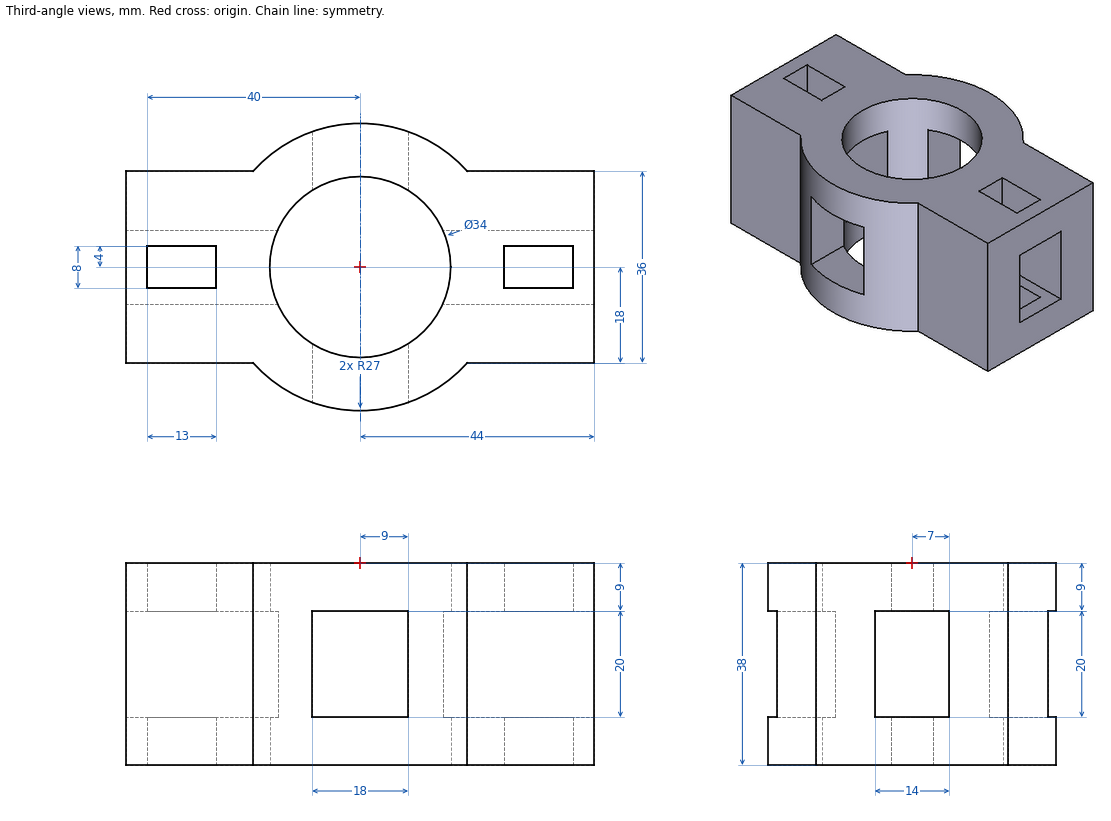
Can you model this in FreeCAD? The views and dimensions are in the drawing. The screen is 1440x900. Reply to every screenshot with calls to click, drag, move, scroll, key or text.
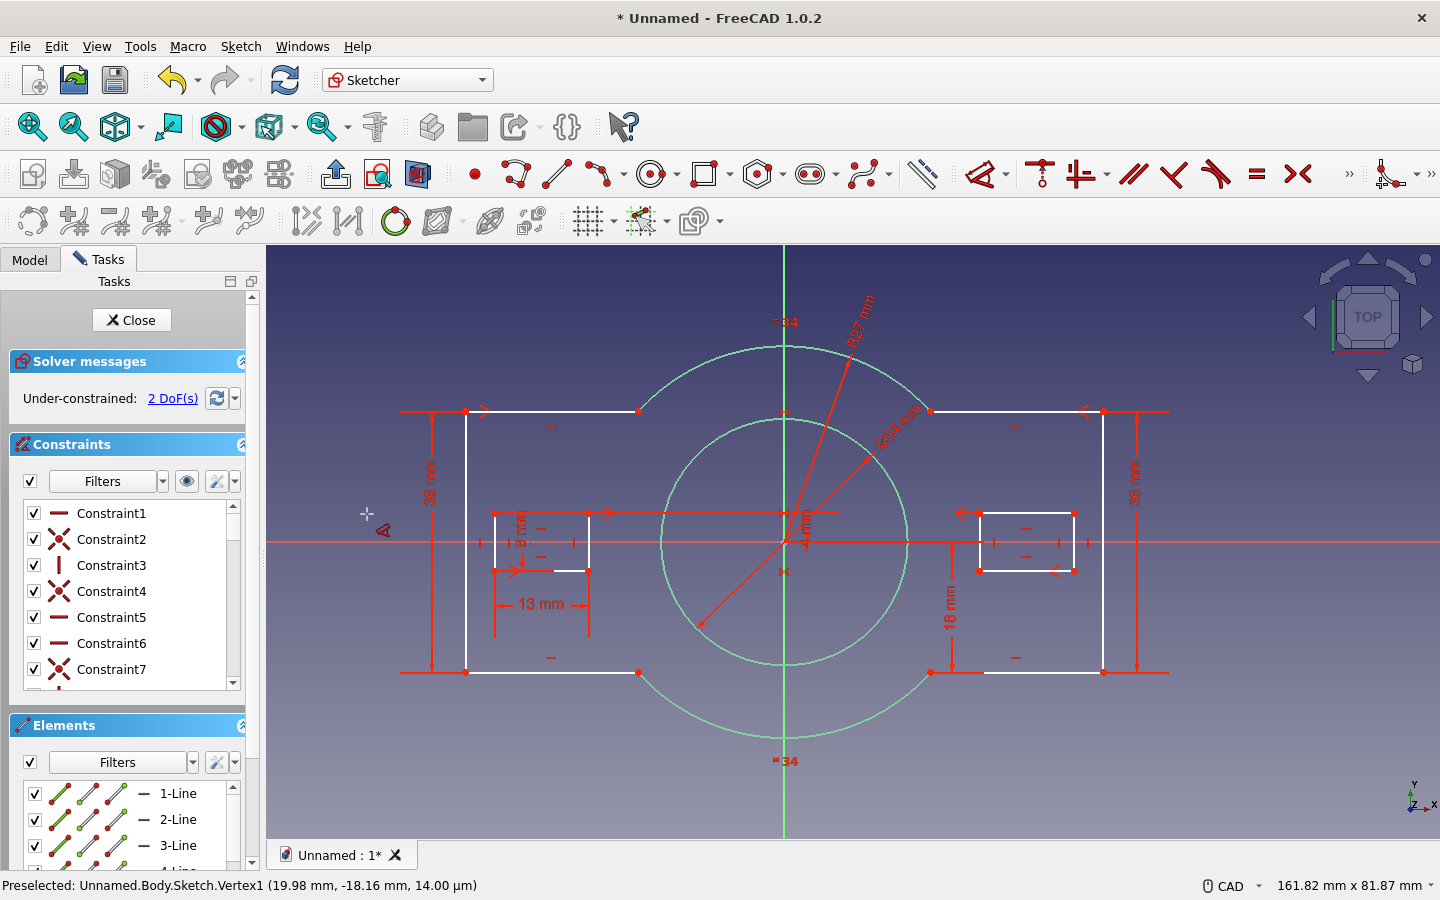
click(1103, 673)
click(944, 707)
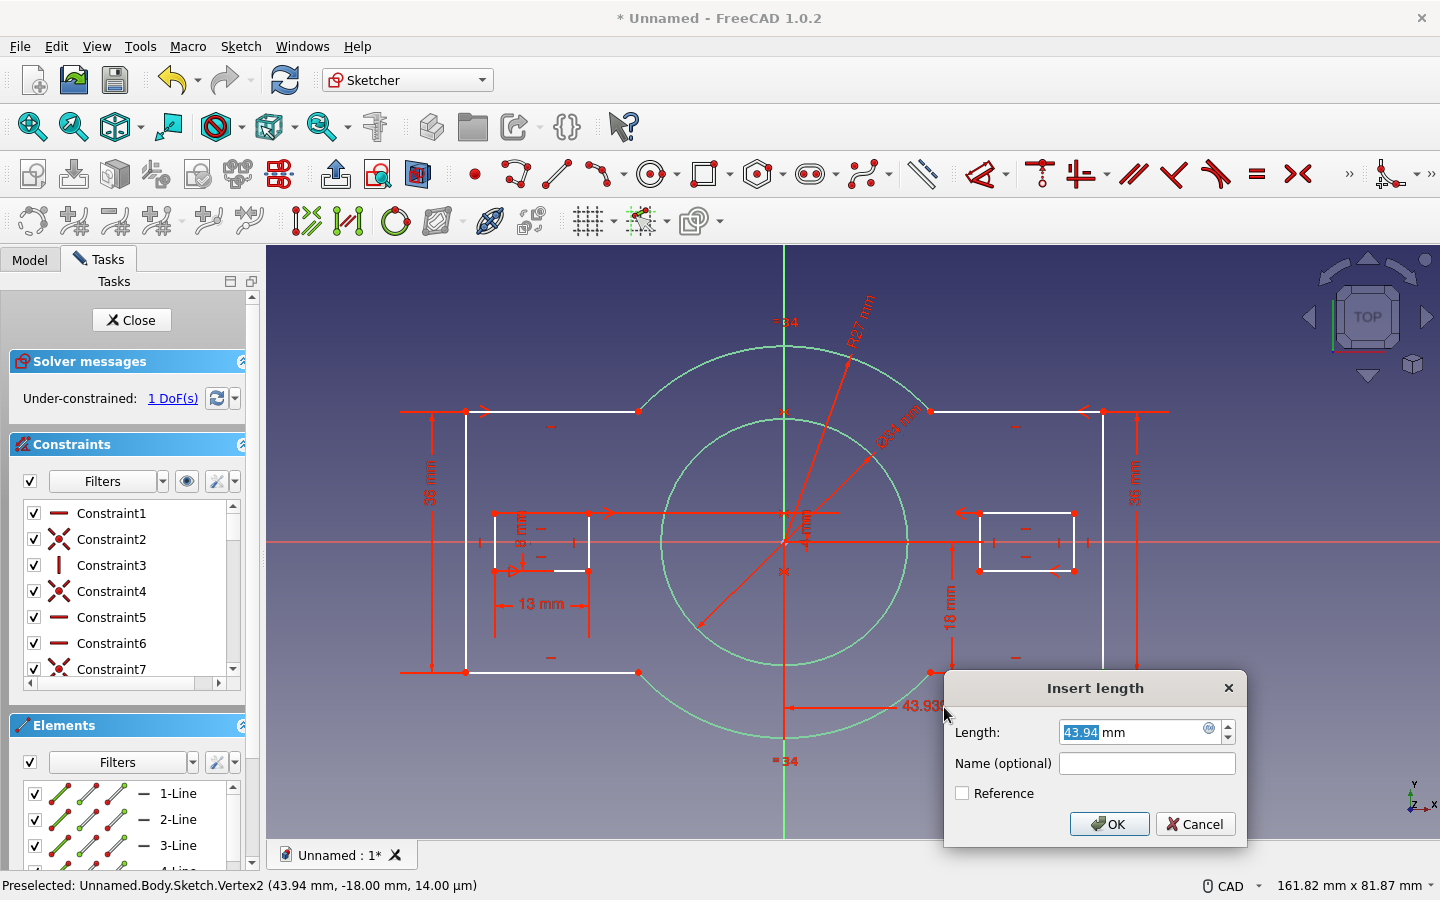
text(44)
key(Return)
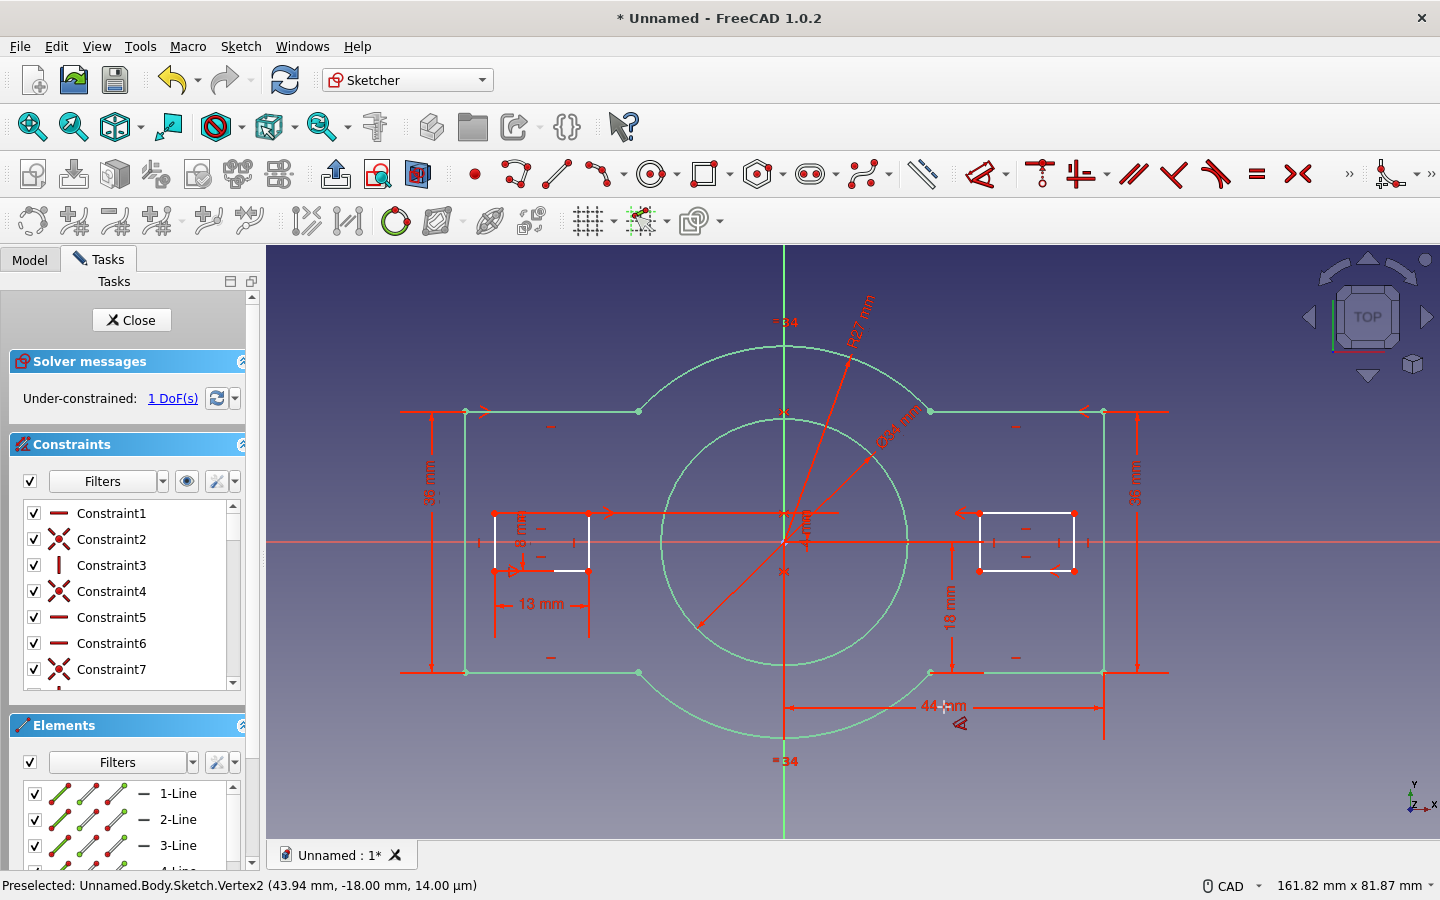
click(495, 513)
click(639, 479)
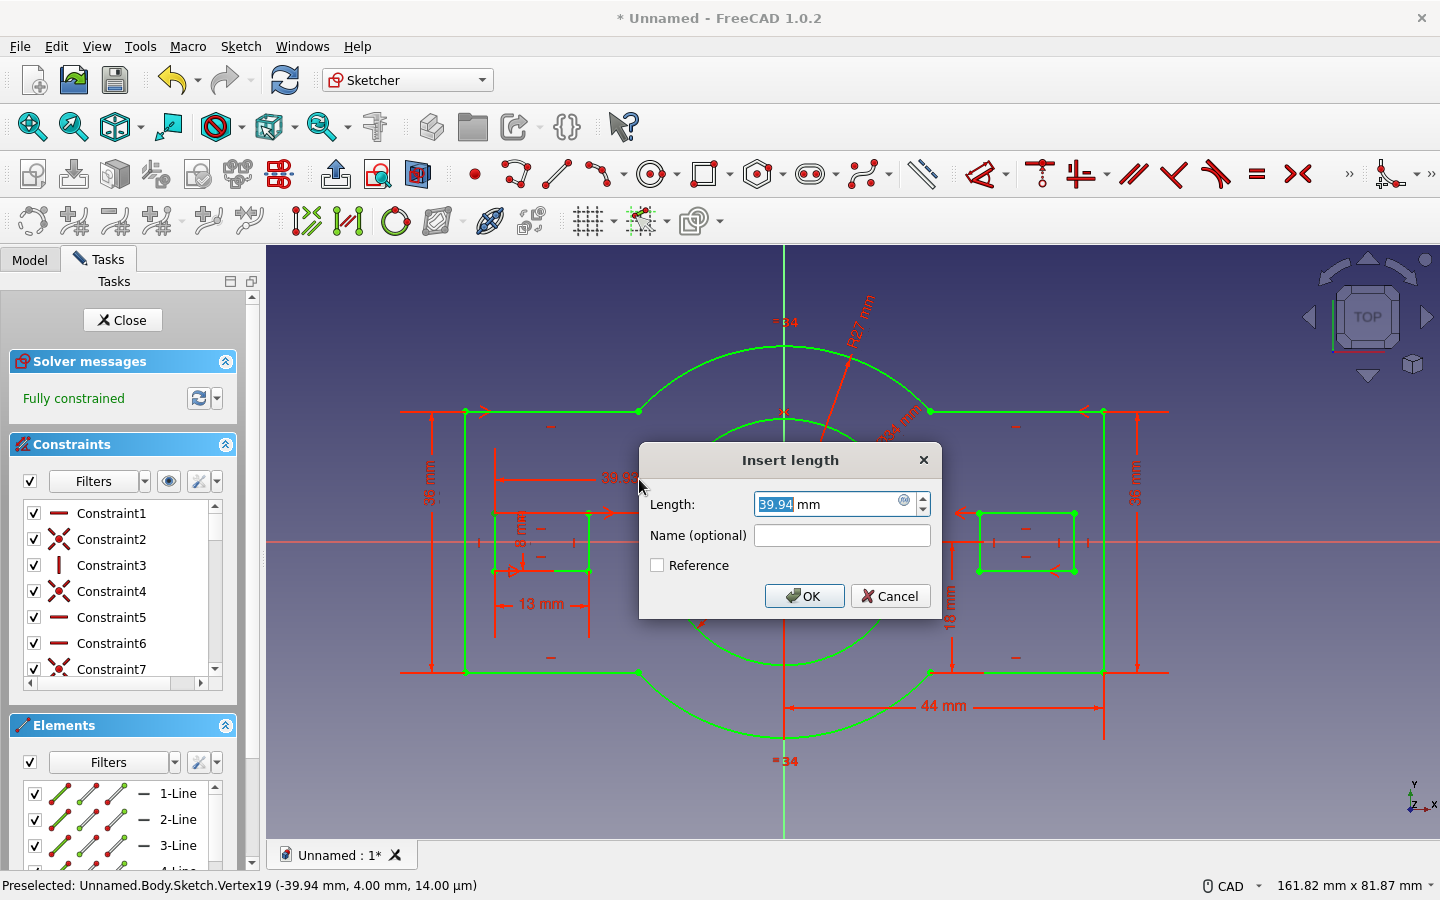
text(40)
key(Return)
key(Escape)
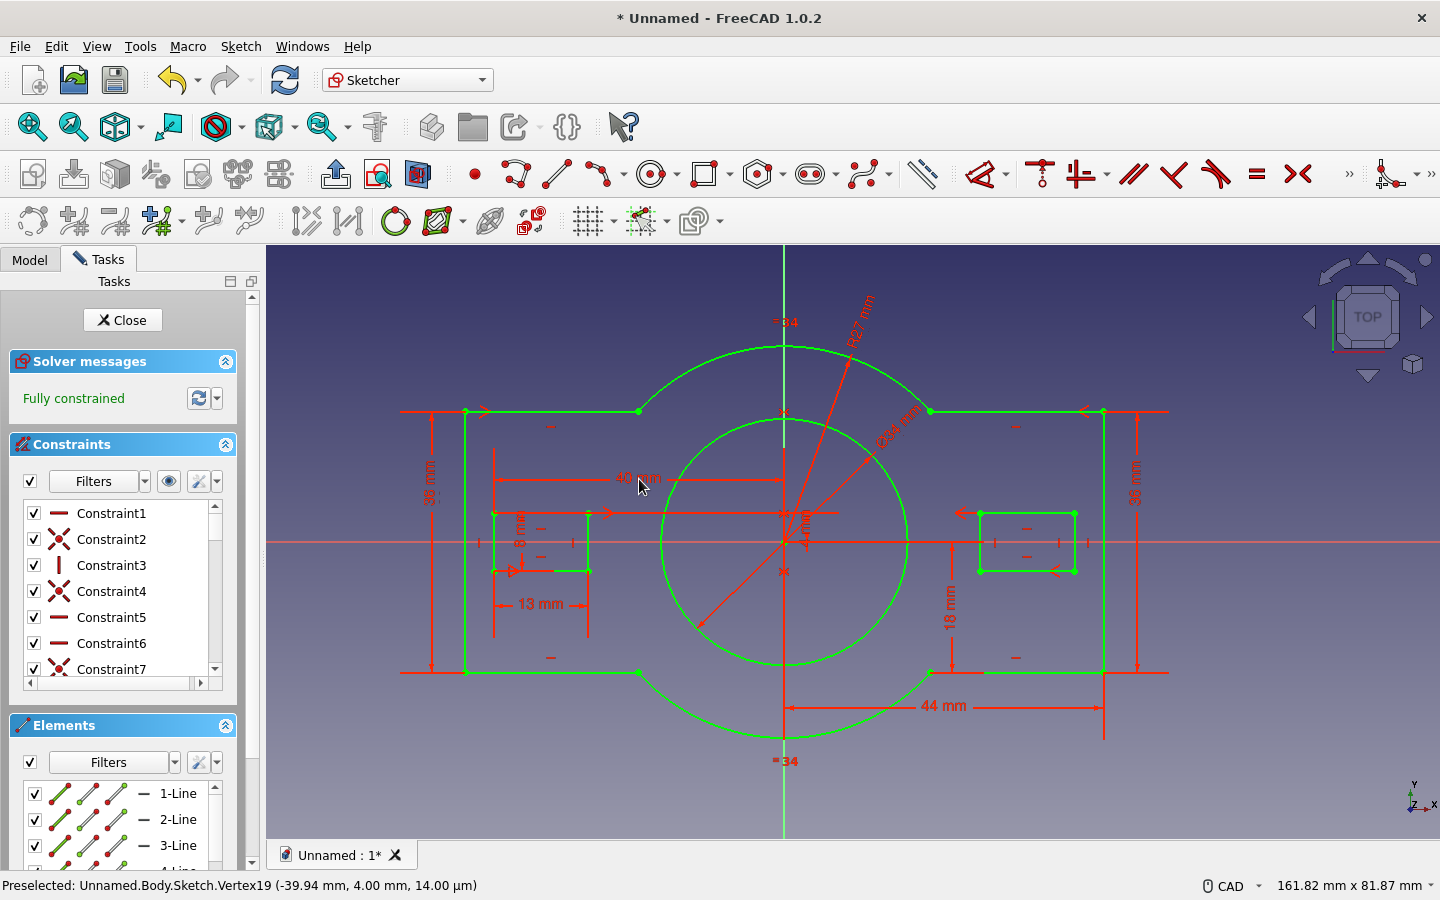
click(123, 320)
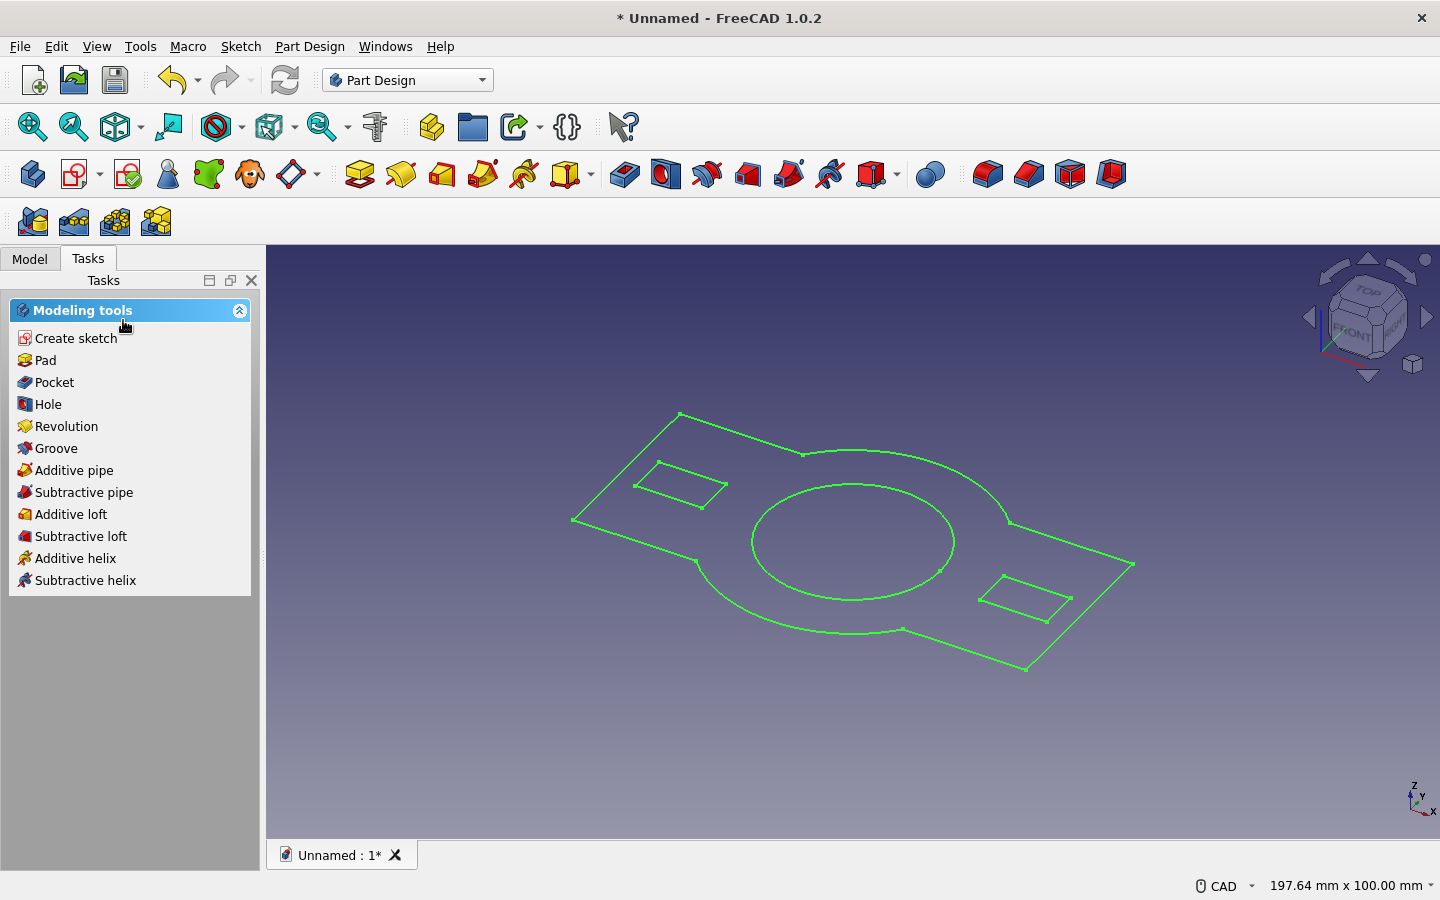
click(360, 174)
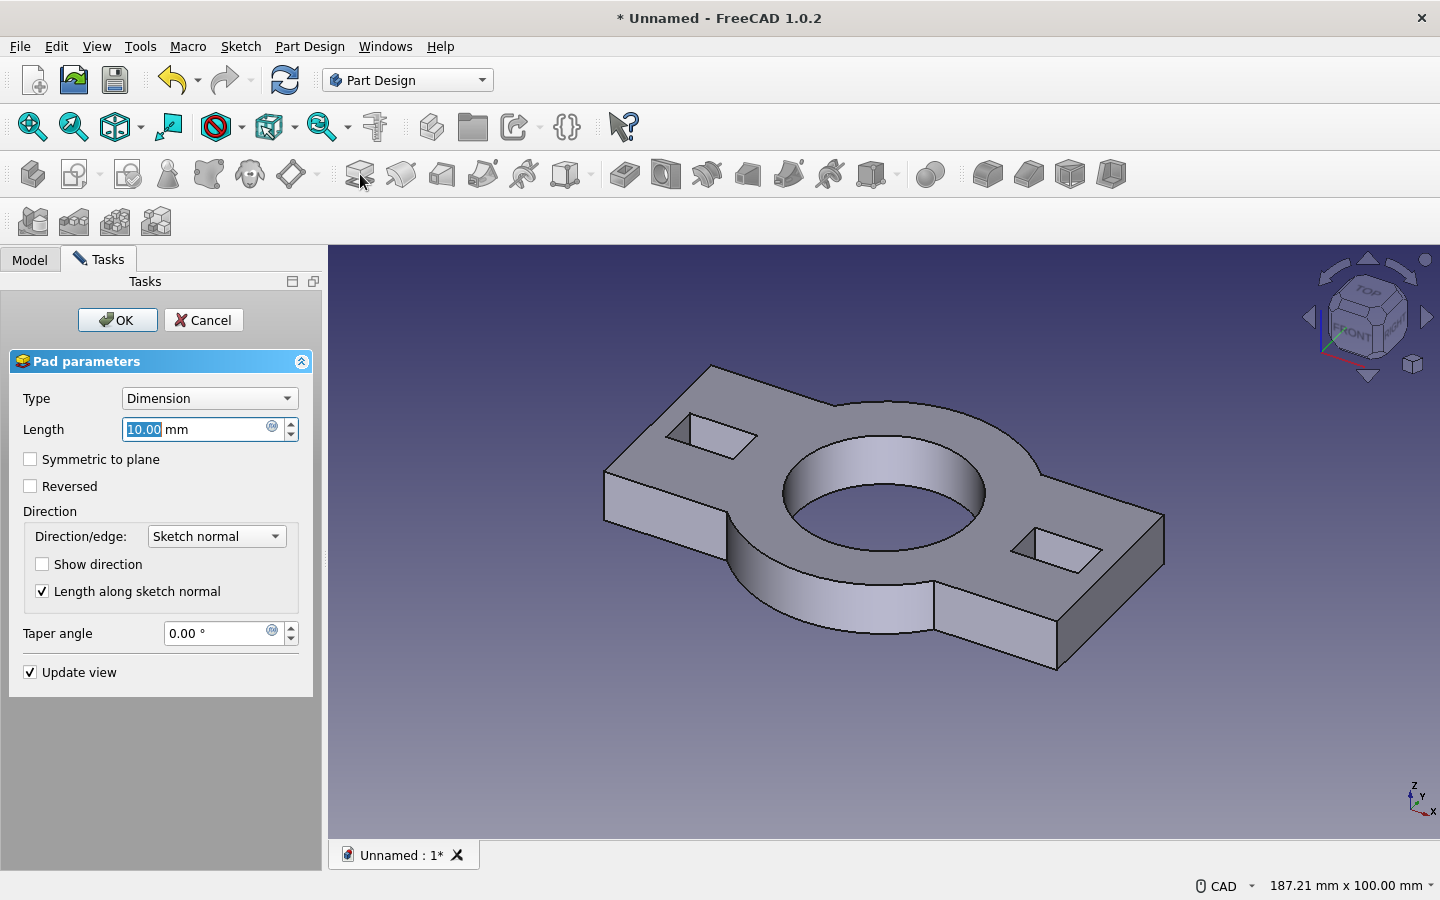
text(38)
key(Tab)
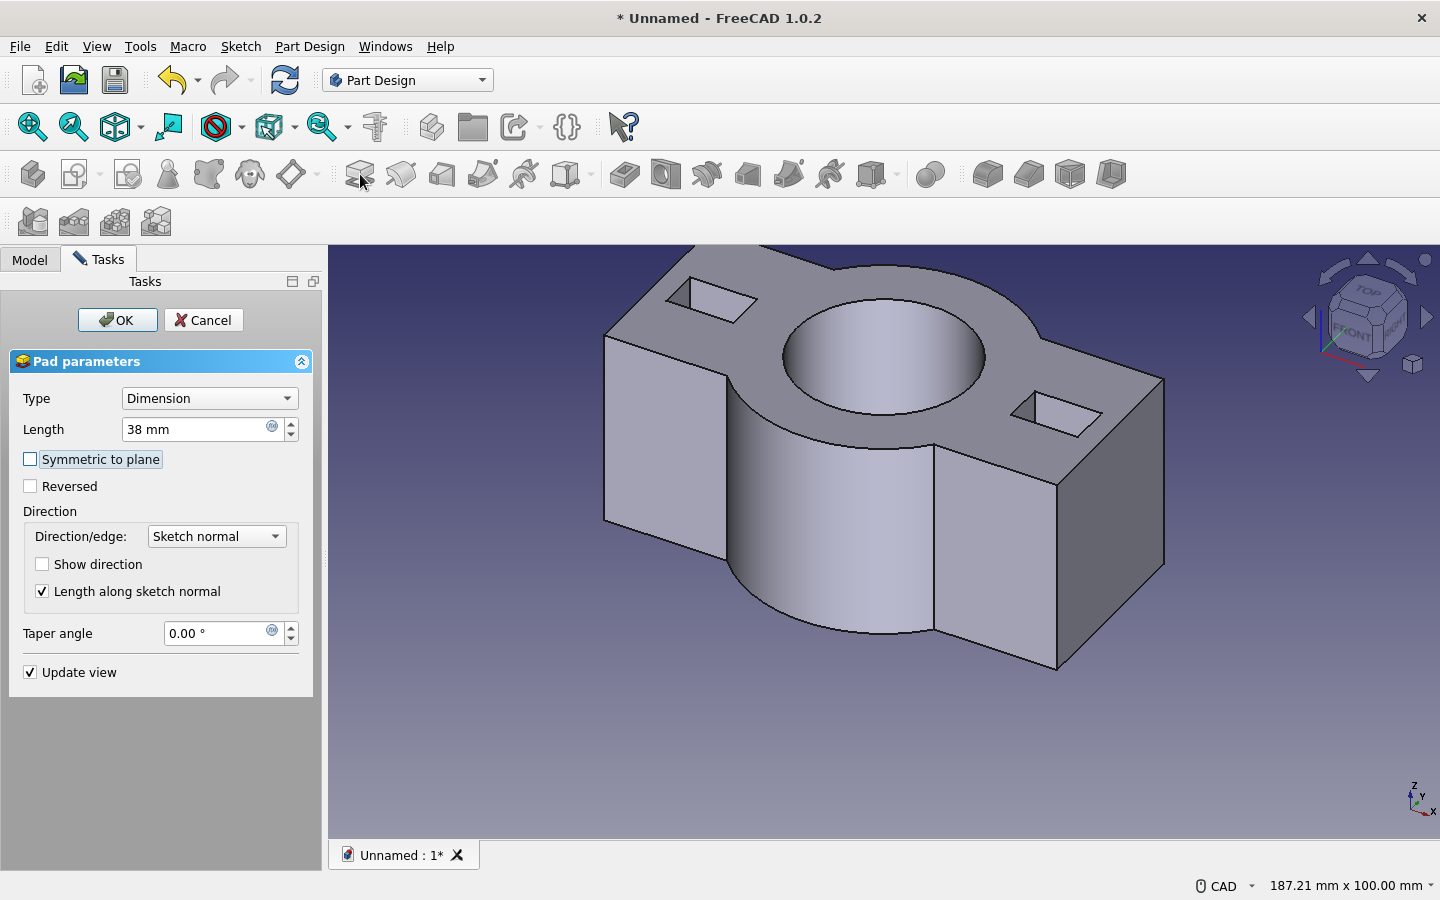
click(31, 486)